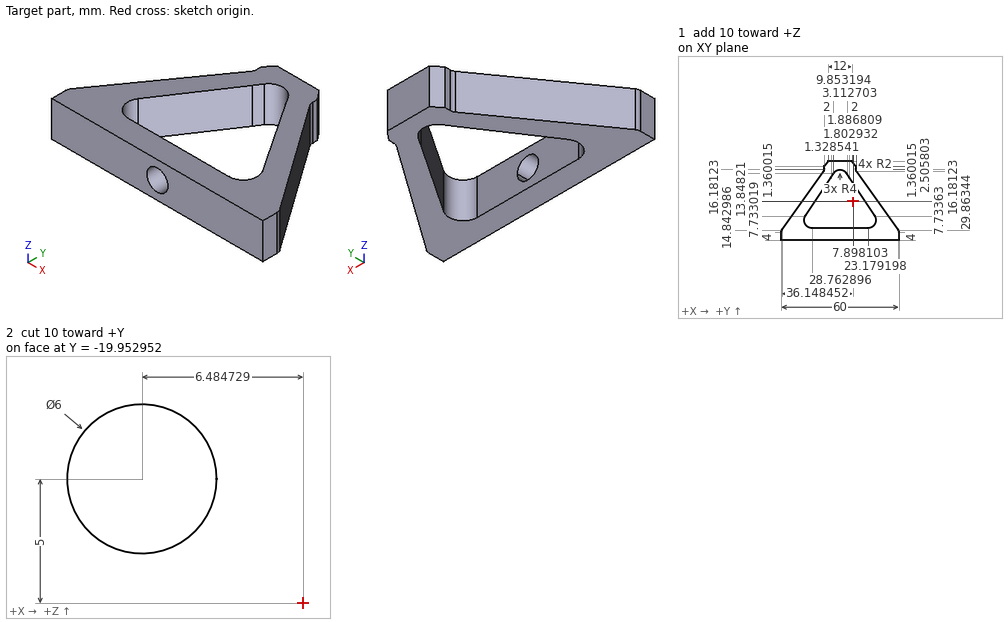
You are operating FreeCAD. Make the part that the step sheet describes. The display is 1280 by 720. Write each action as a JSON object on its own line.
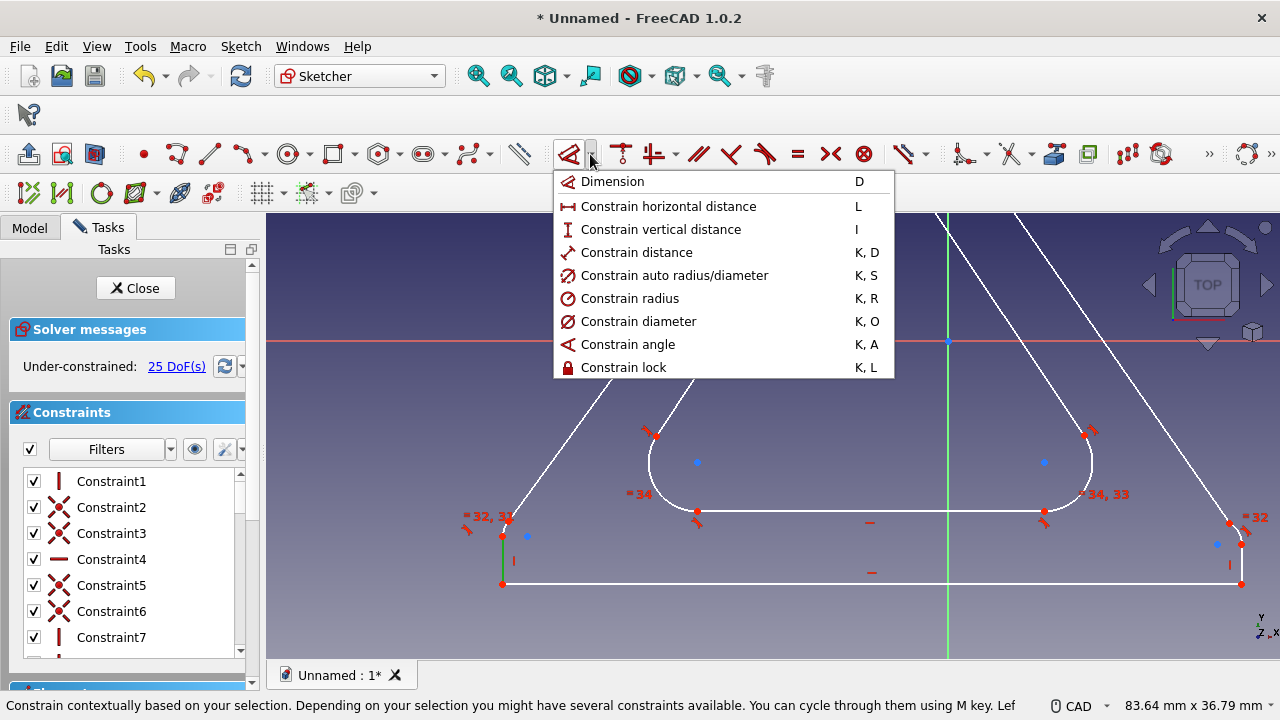
{"action": "left_click", "coordinate": [724, 230]}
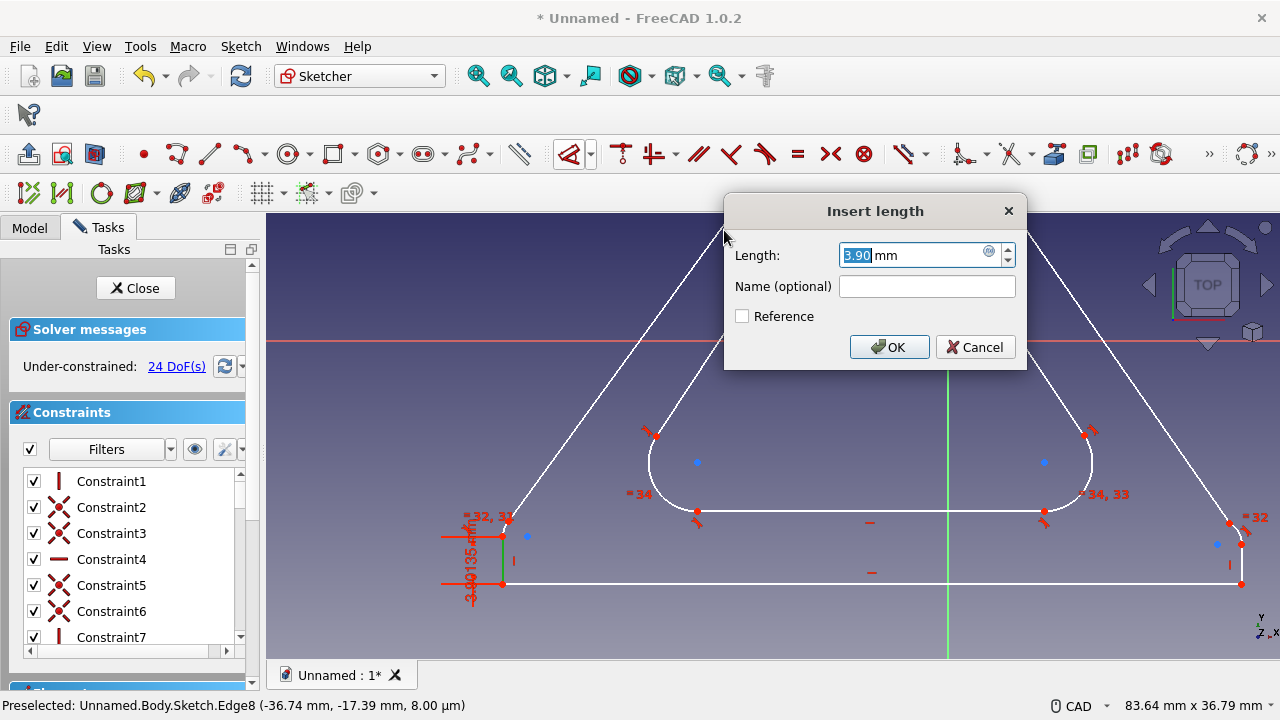
{"action": "type", "text": "4"}
{"action": "key", "text": "Return"}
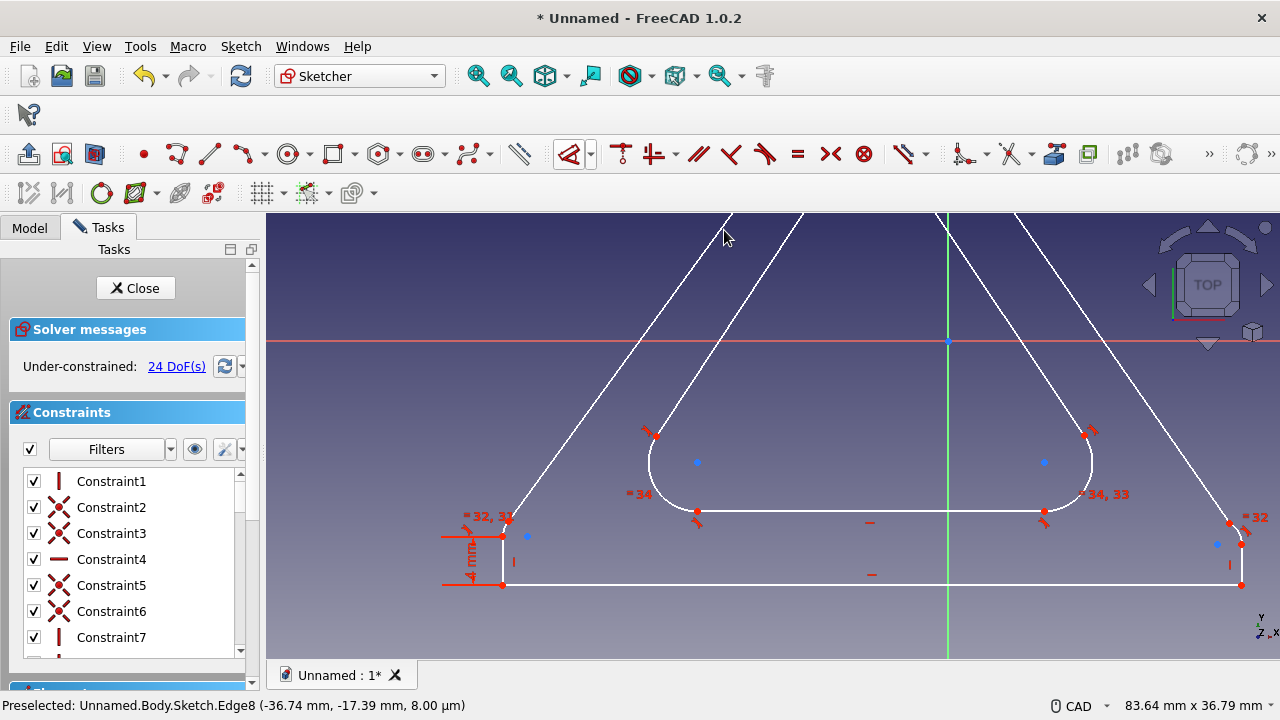
{"action": "scroll", "coordinate": [503, 552], "scroll_direction": "down", "scroll_amount": 3}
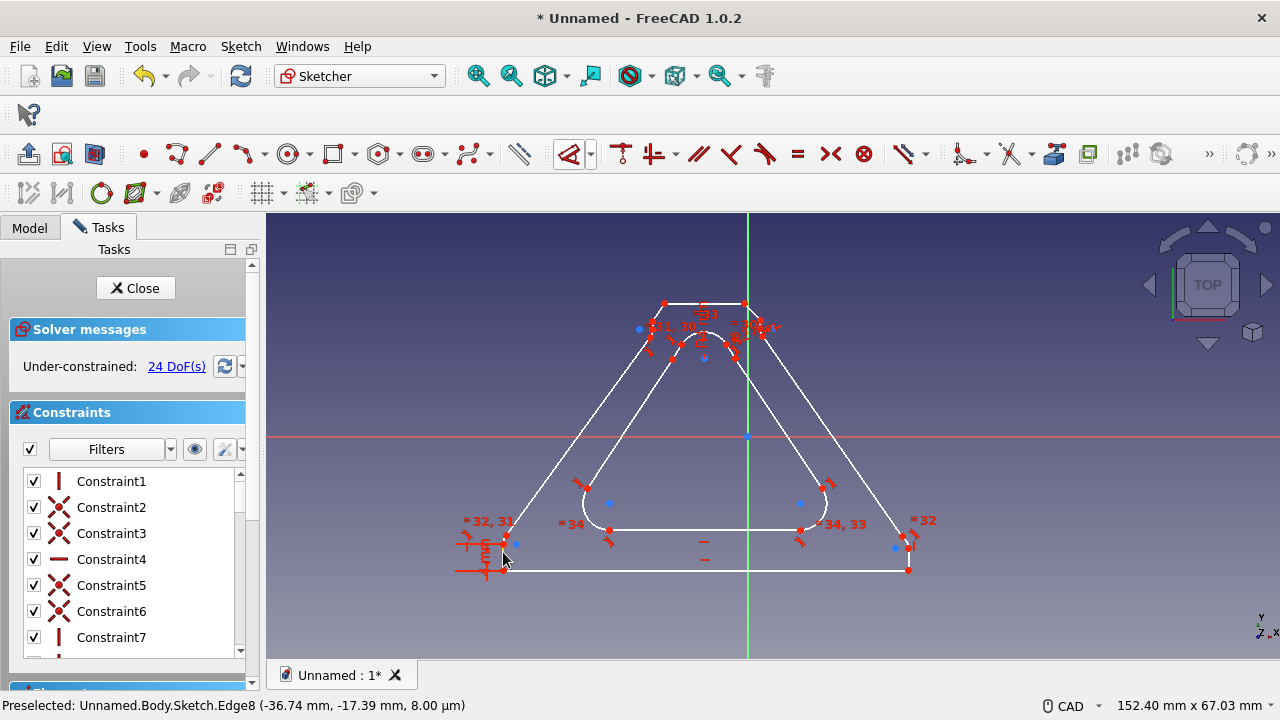
{"action": "scroll", "coordinate": [909, 564], "scroll_direction": "up", "scroll_amount": 4}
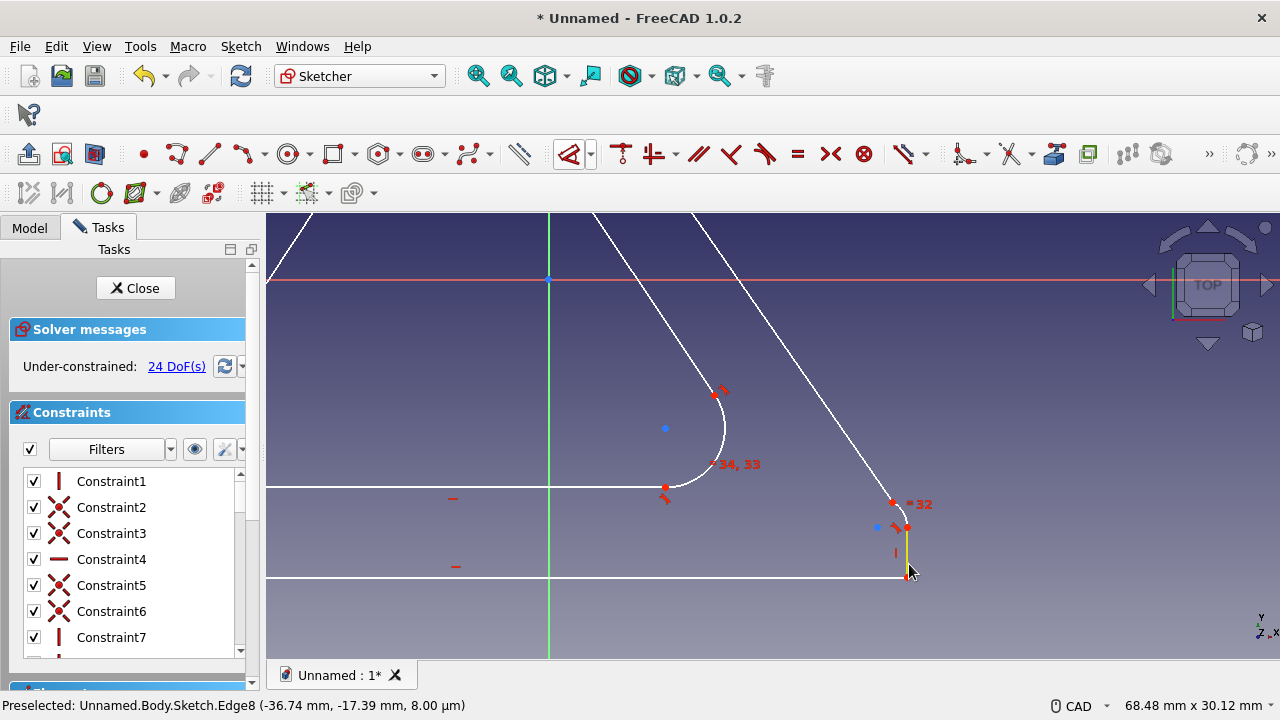
{"action": "left_click", "coordinate": [907, 563]}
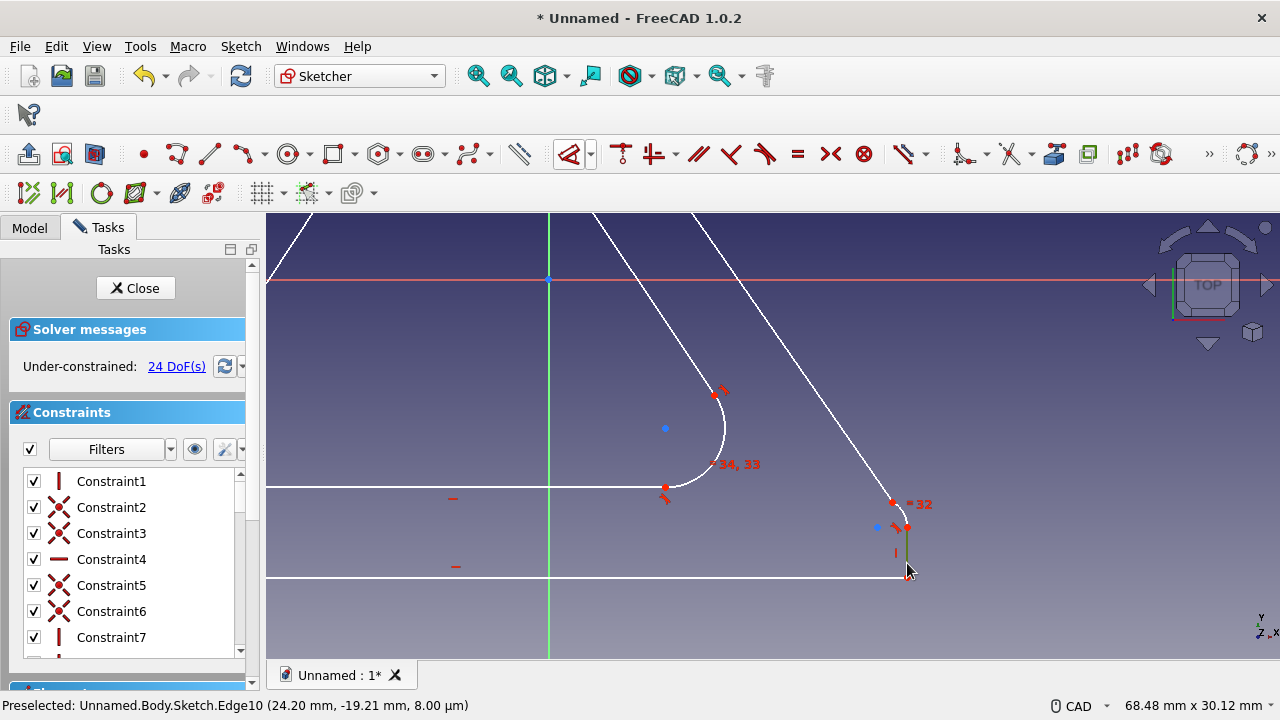
{"action": "left_click", "coordinate": [590, 154]}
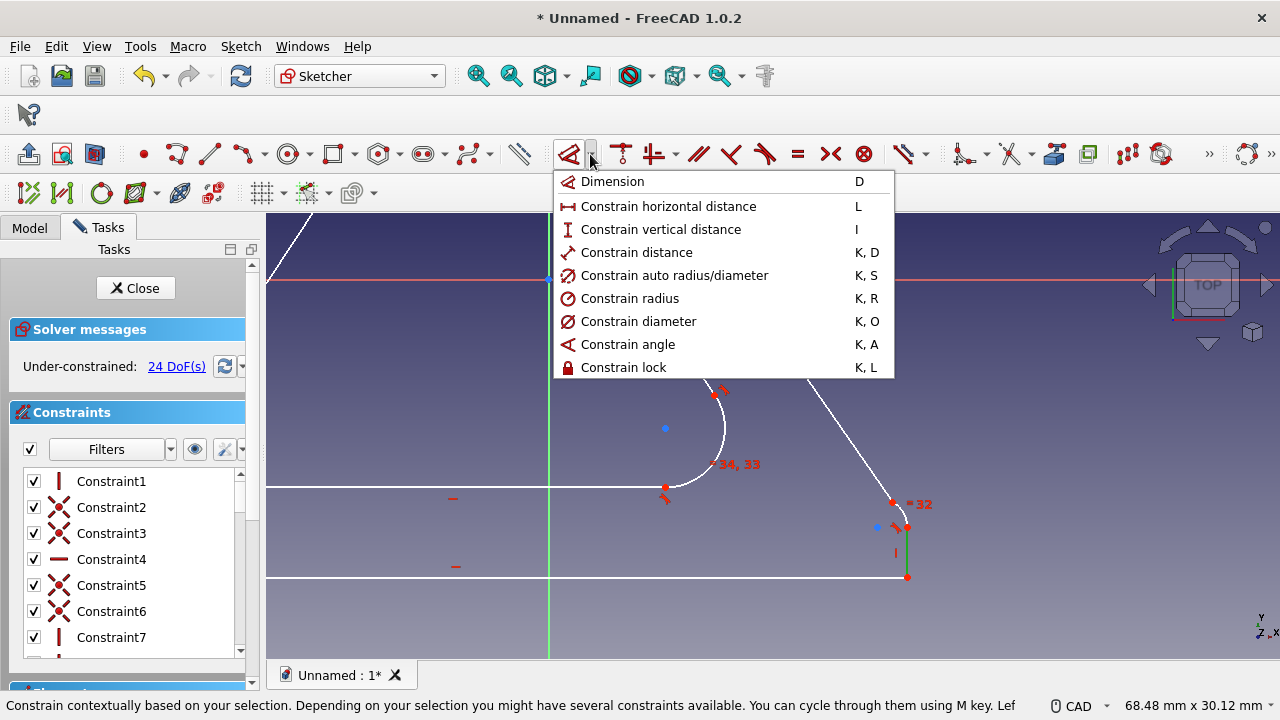
{"action": "left_click", "coordinate": [724, 230]}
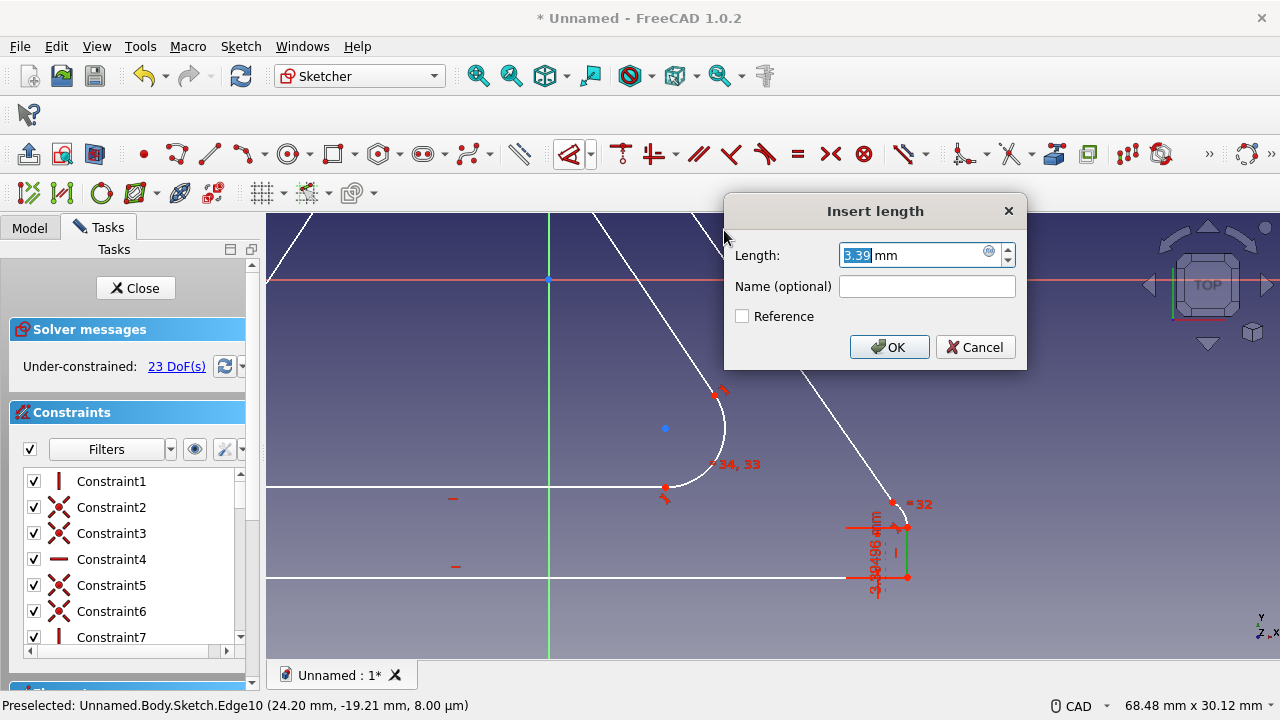
{"action": "type", "text": "4"}
{"action": "key", "text": "Return"}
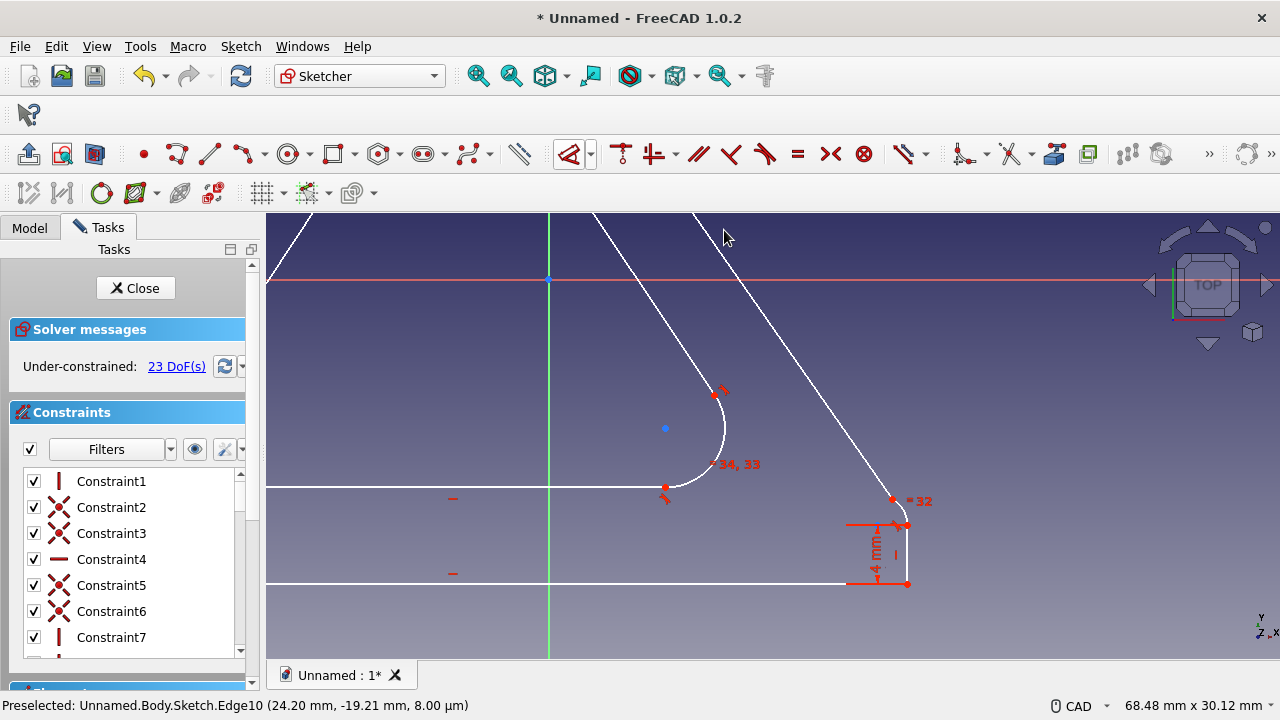
{"action": "scroll", "coordinate": [910, 564], "scroll_direction": "down", "scroll_amount": 4}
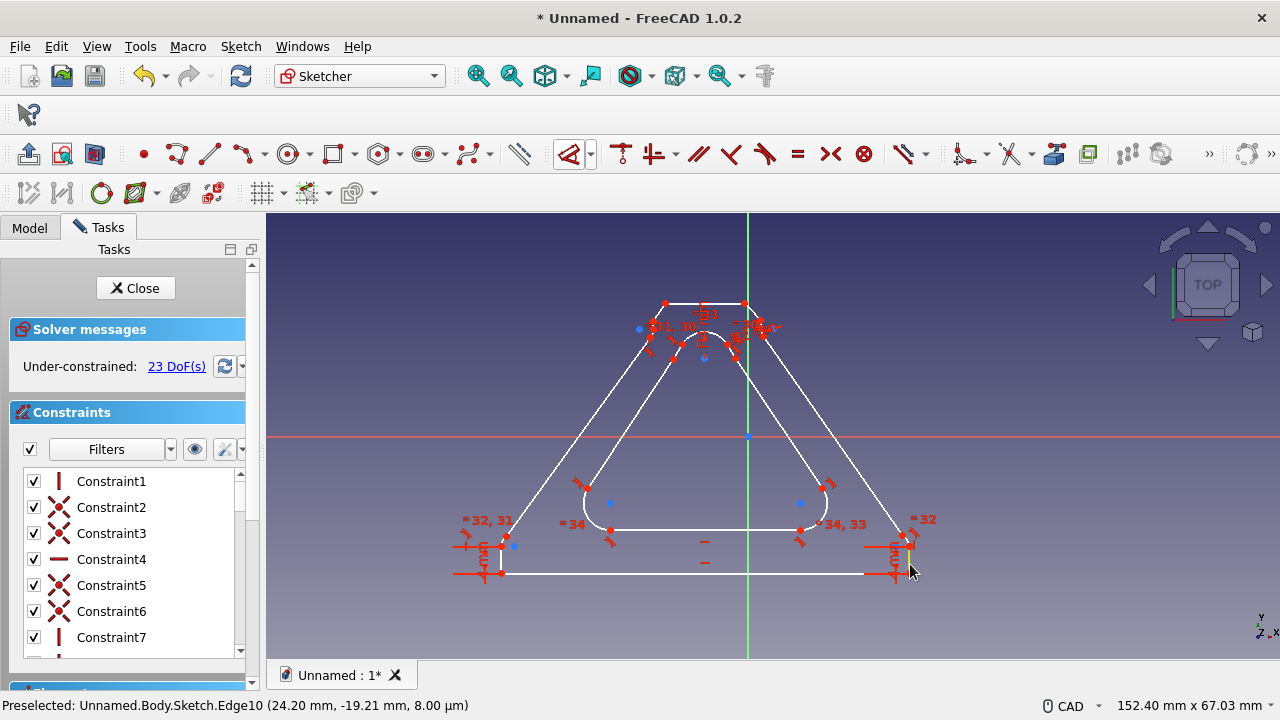
{"action": "left_click", "coordinate": [721, 304]}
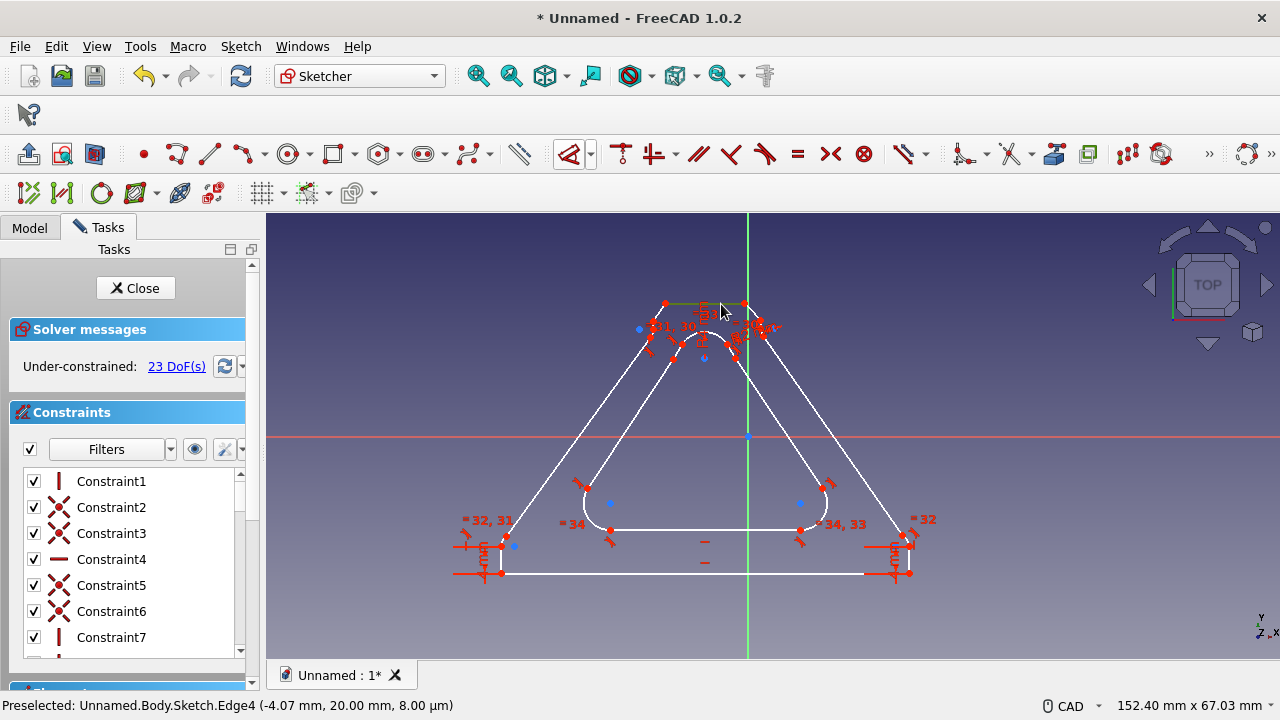
{"action": "left_click", "coordinate": [590, 154]}